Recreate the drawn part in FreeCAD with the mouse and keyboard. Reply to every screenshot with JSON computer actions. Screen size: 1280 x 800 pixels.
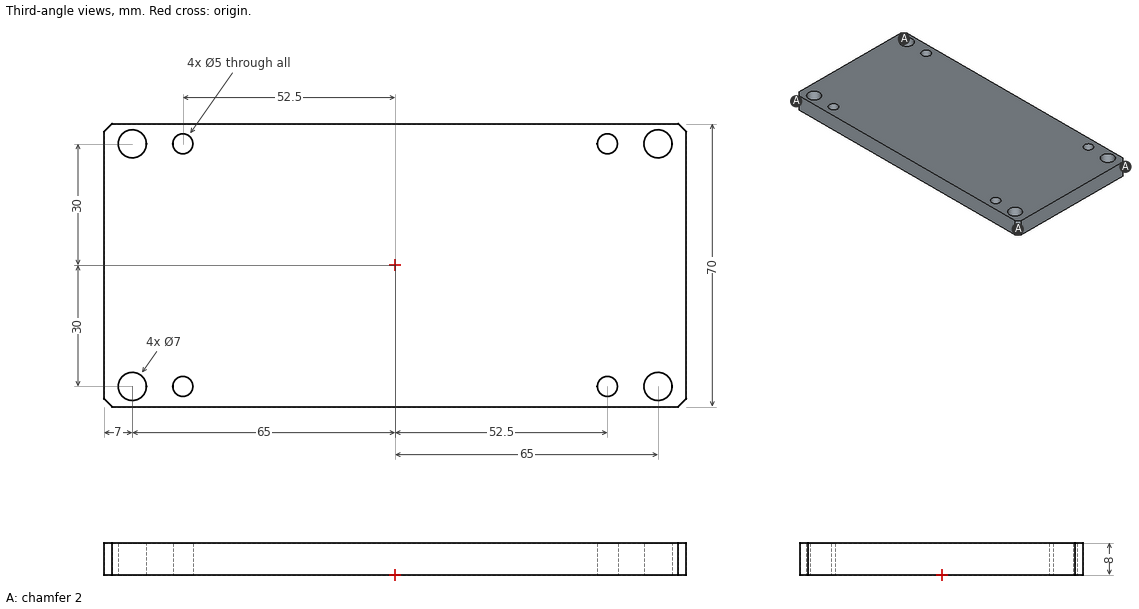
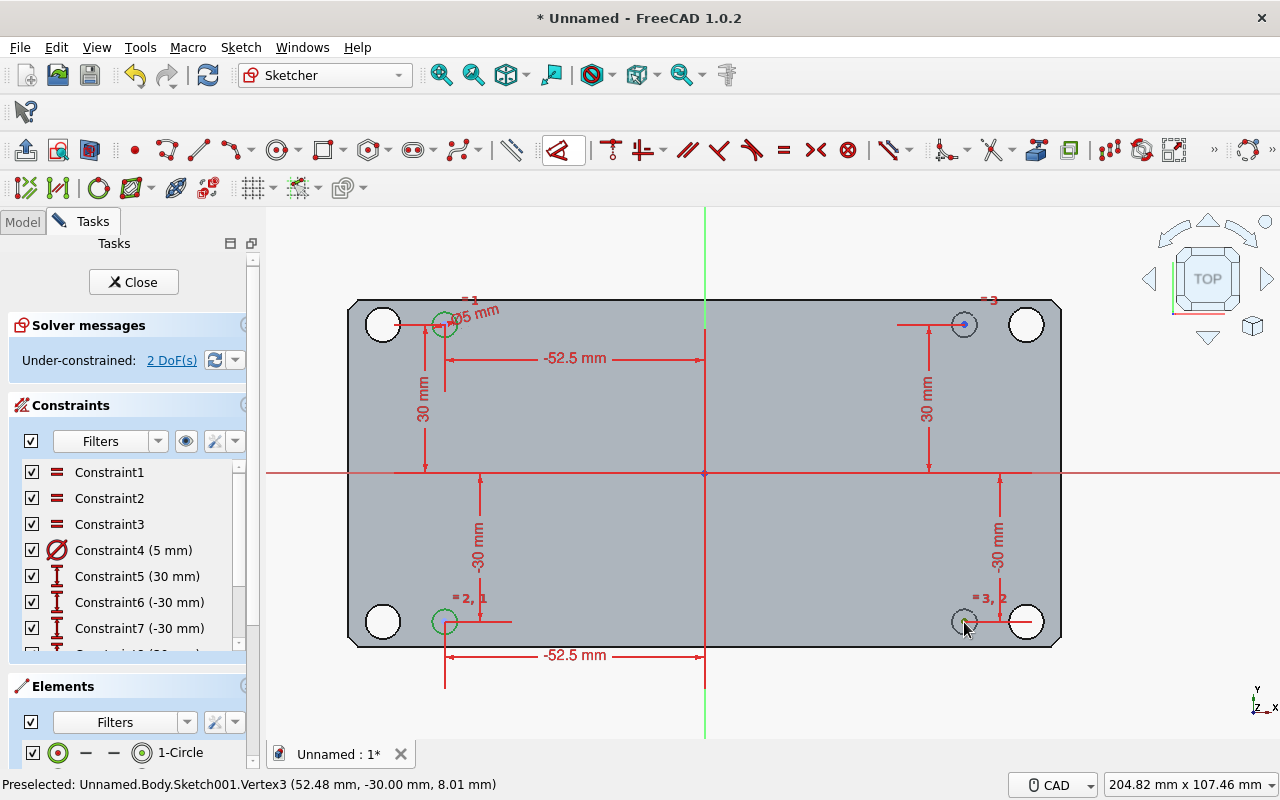
{"action": "key", "text": "l"}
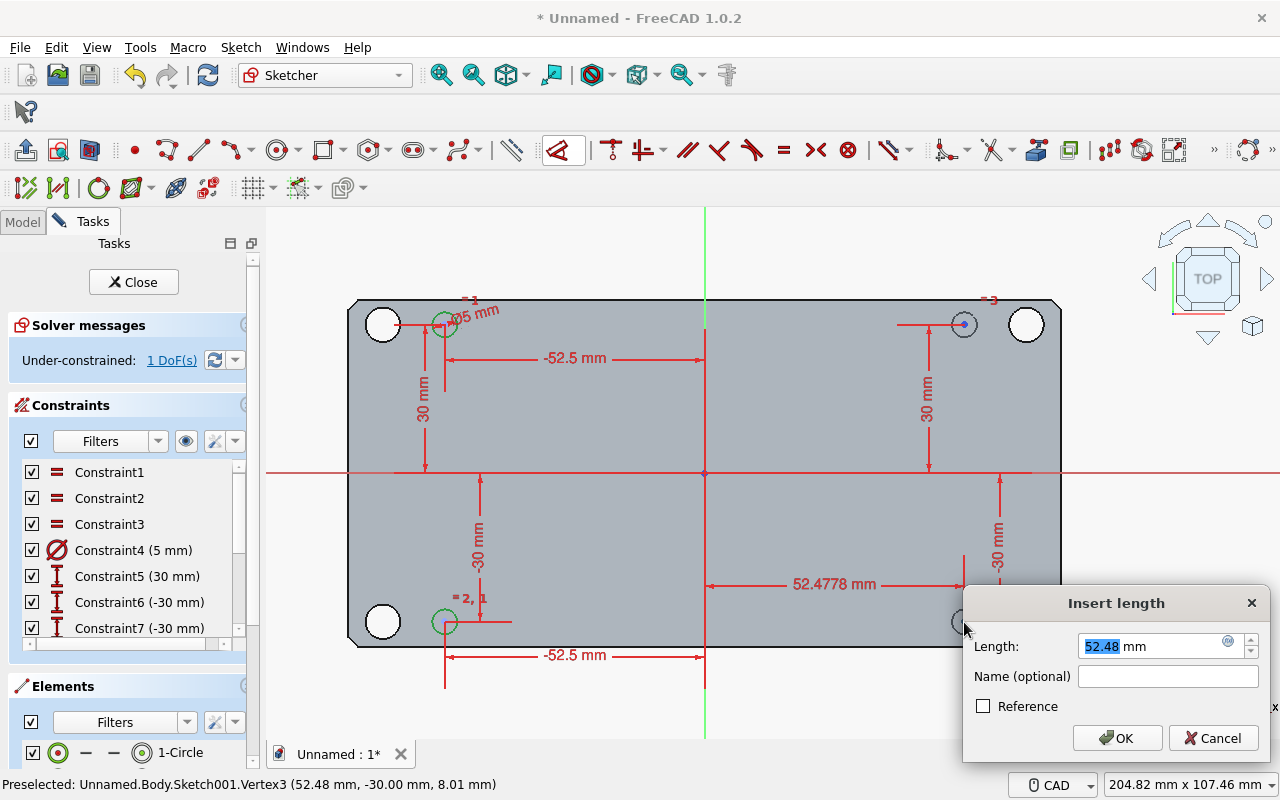
{"action": "type", "text": "52.5"}
{"action": "key", "text": "Return"}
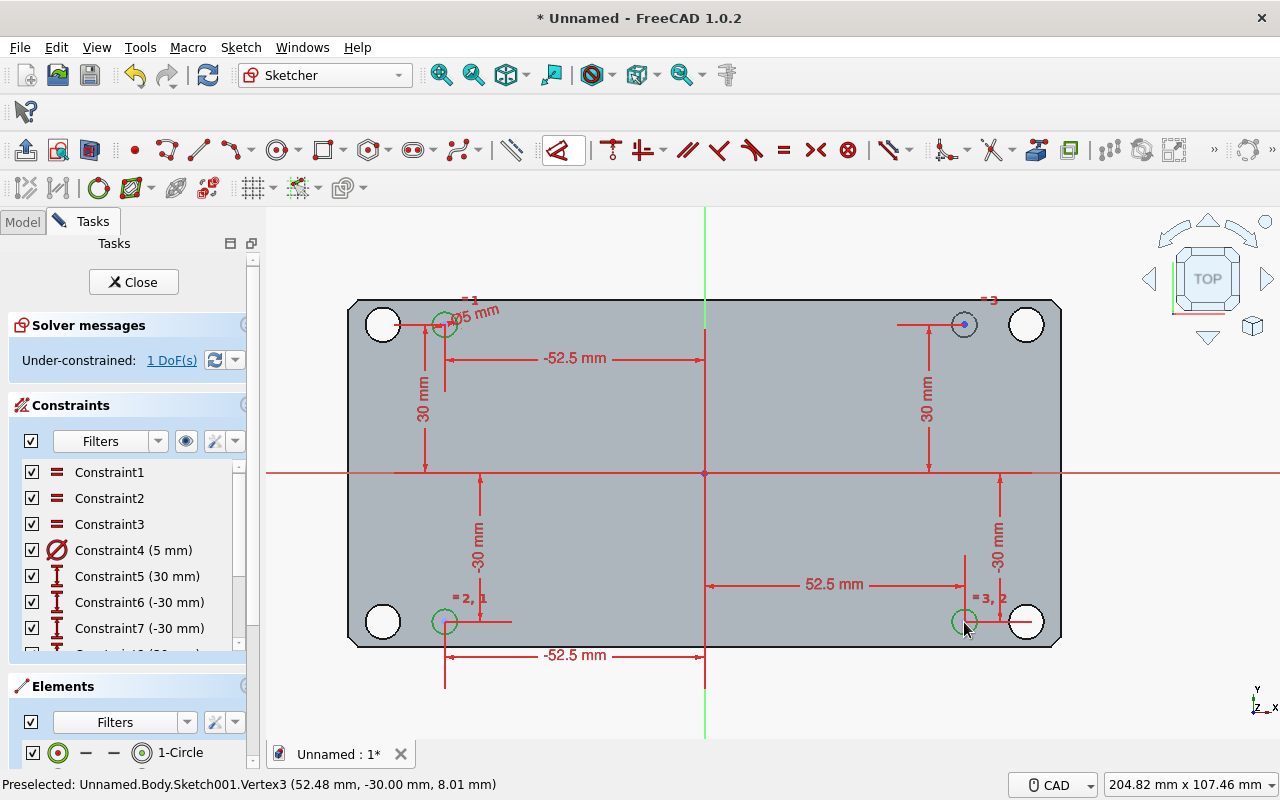
{"action": "left_click", "coordinate": [964, 325]}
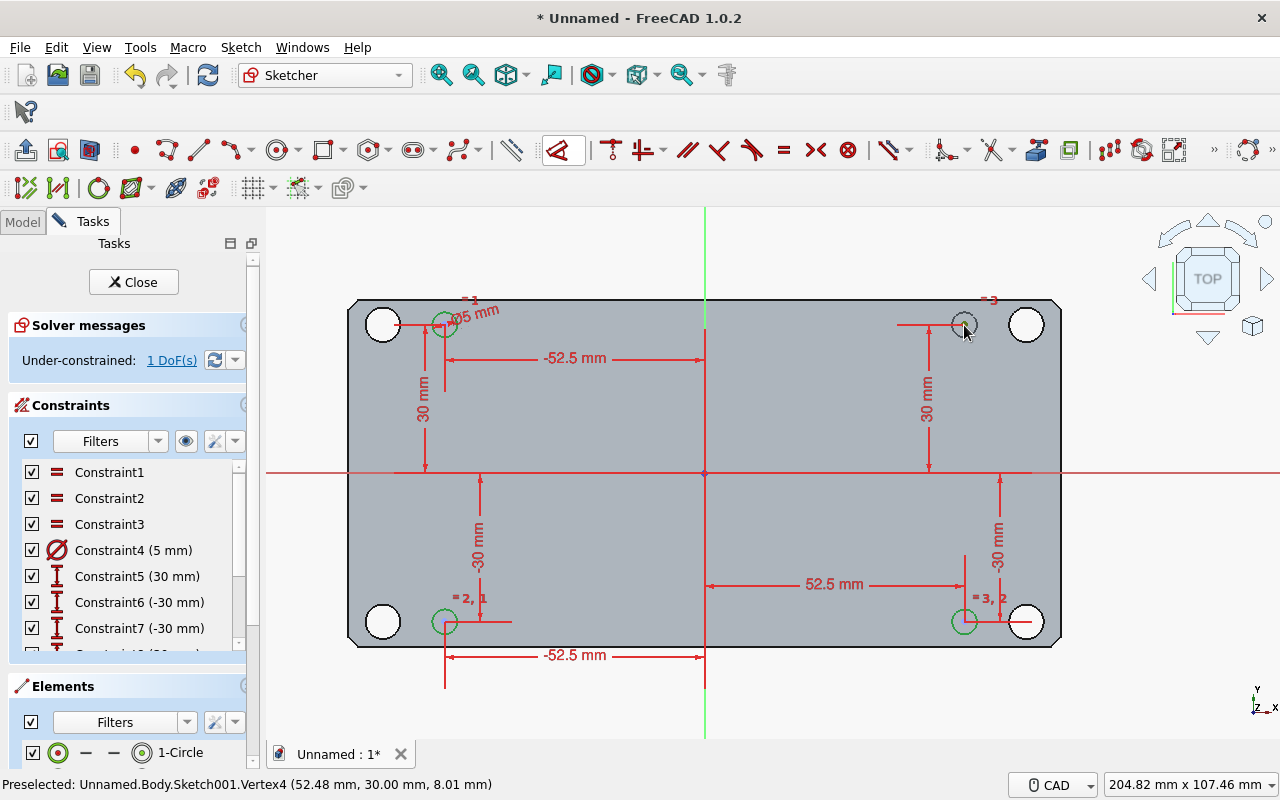
{"action": "left_click", "coordinate": [580, 150]}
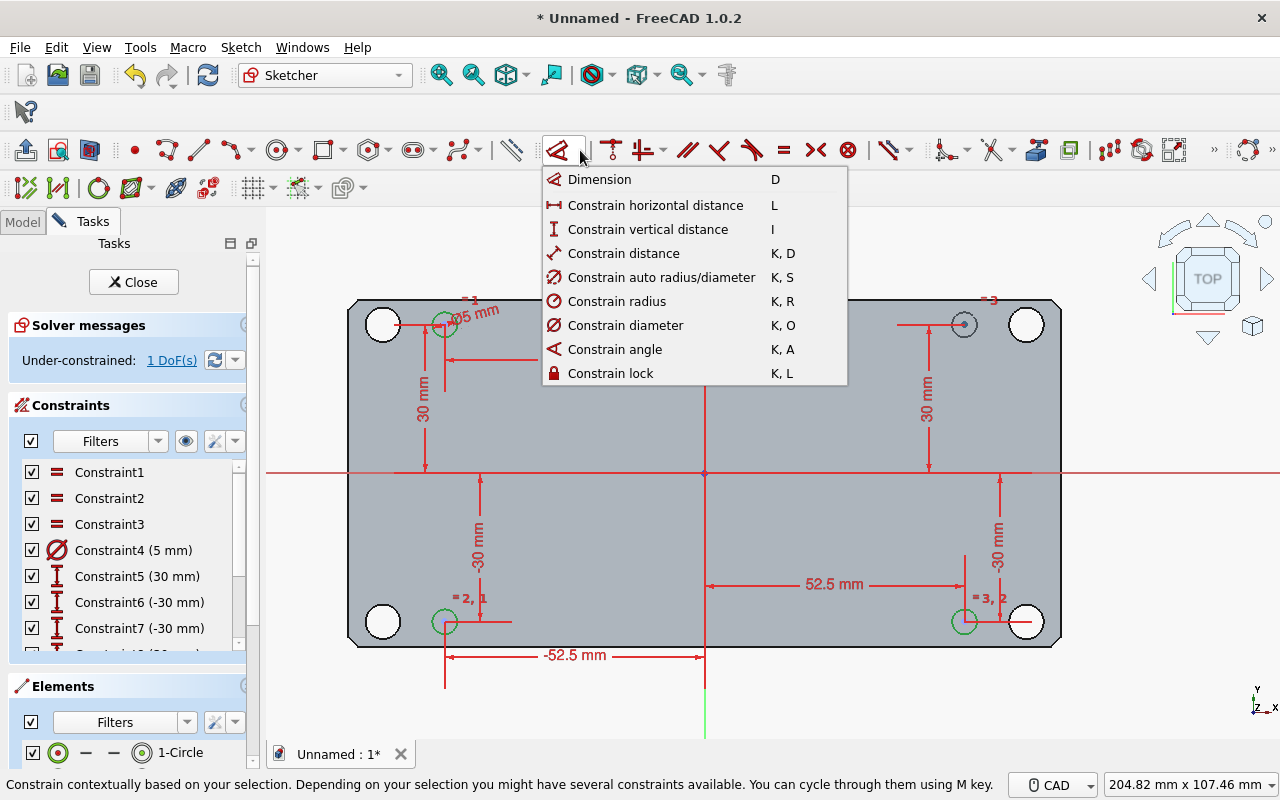
{"action": "left_click", "coordinate": [695, 205]}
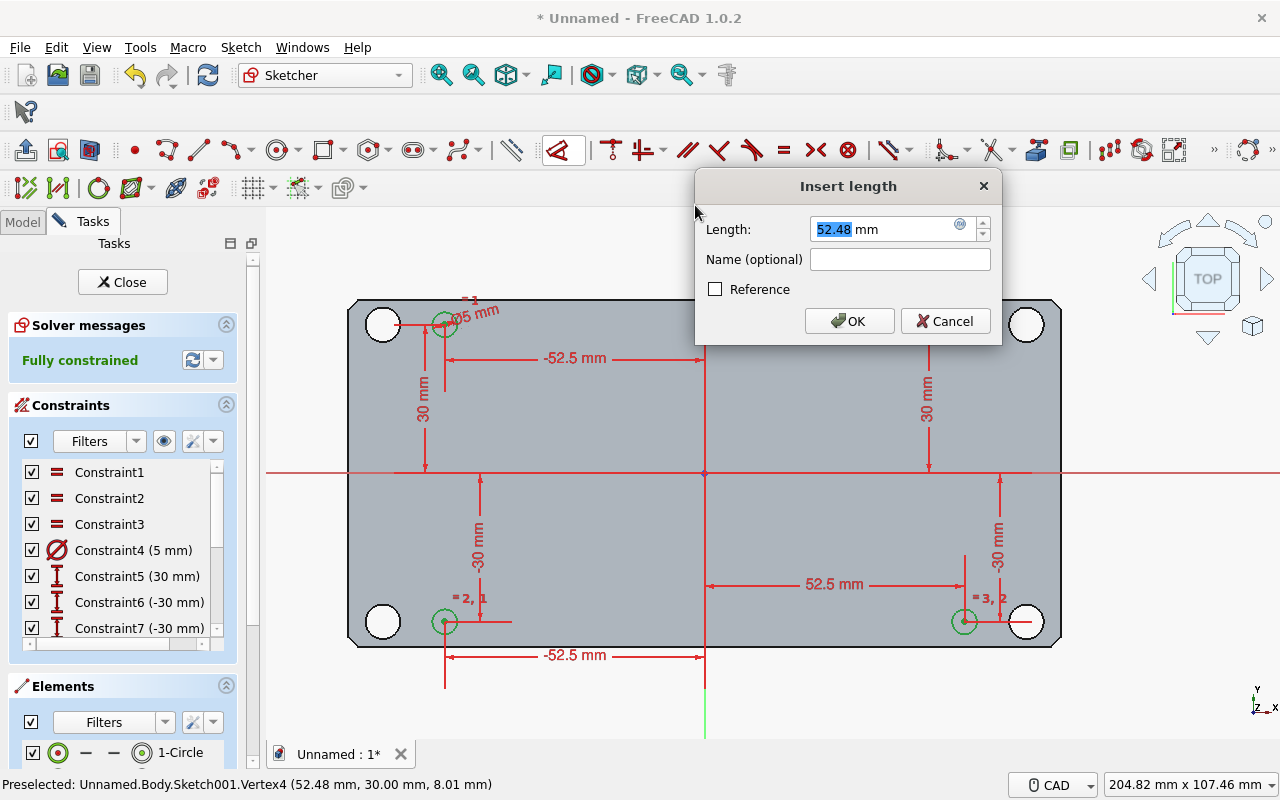
{"action": "type", "text": "52.5"}
{"action": "key", "text": "Return"}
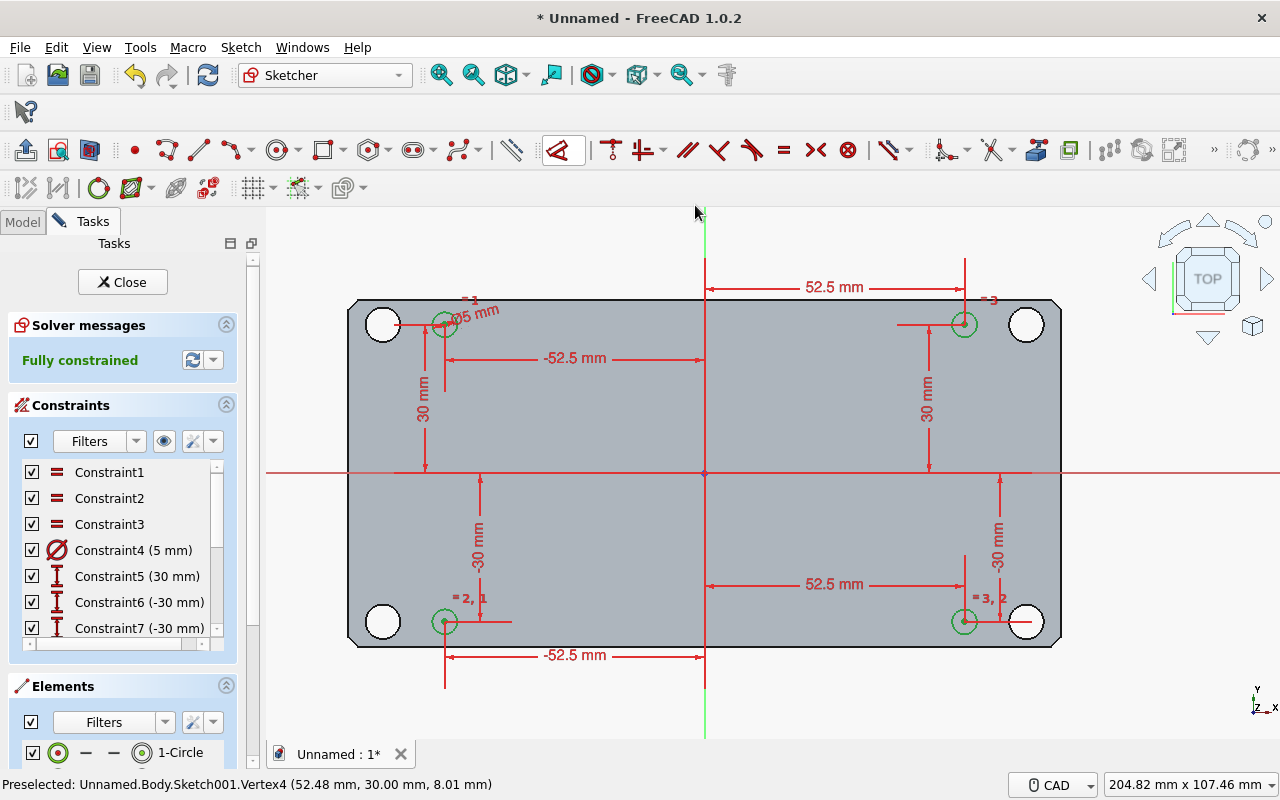
{"action": "left_click", "coordinate": [123, 282]}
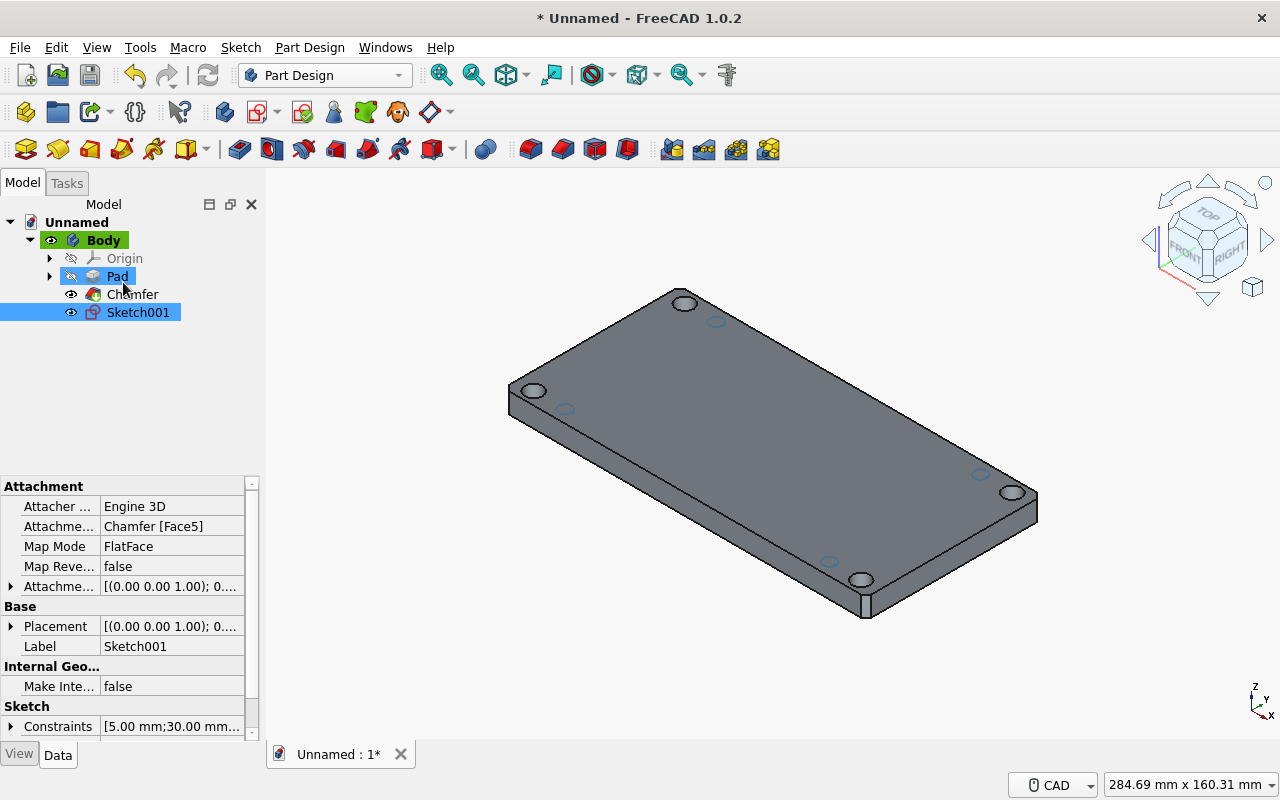
{"action": "left_click", "coordinate": [272, 150]}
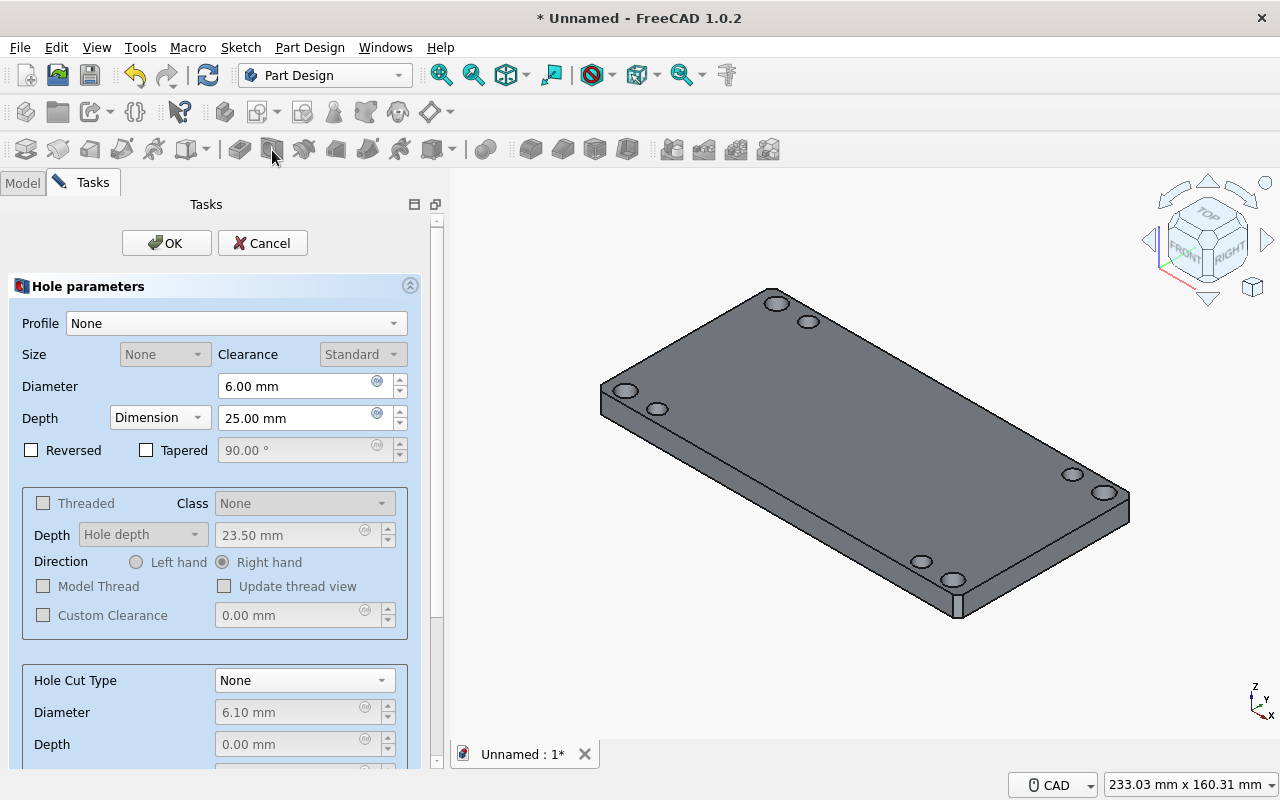
{"action": "triple_click", "coordinate": [305, 386]}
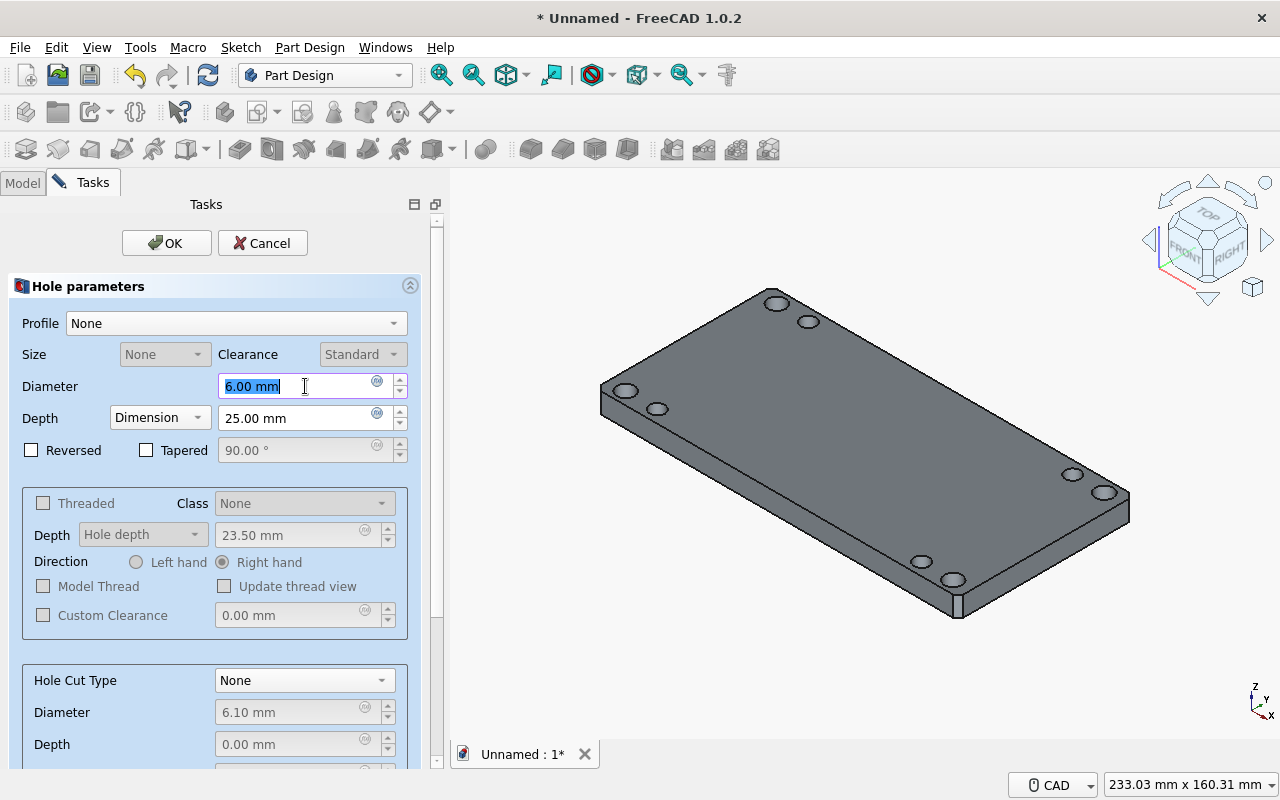
{"action": "type", "text": "5"}
{"action": "key", "text": "Tab"}